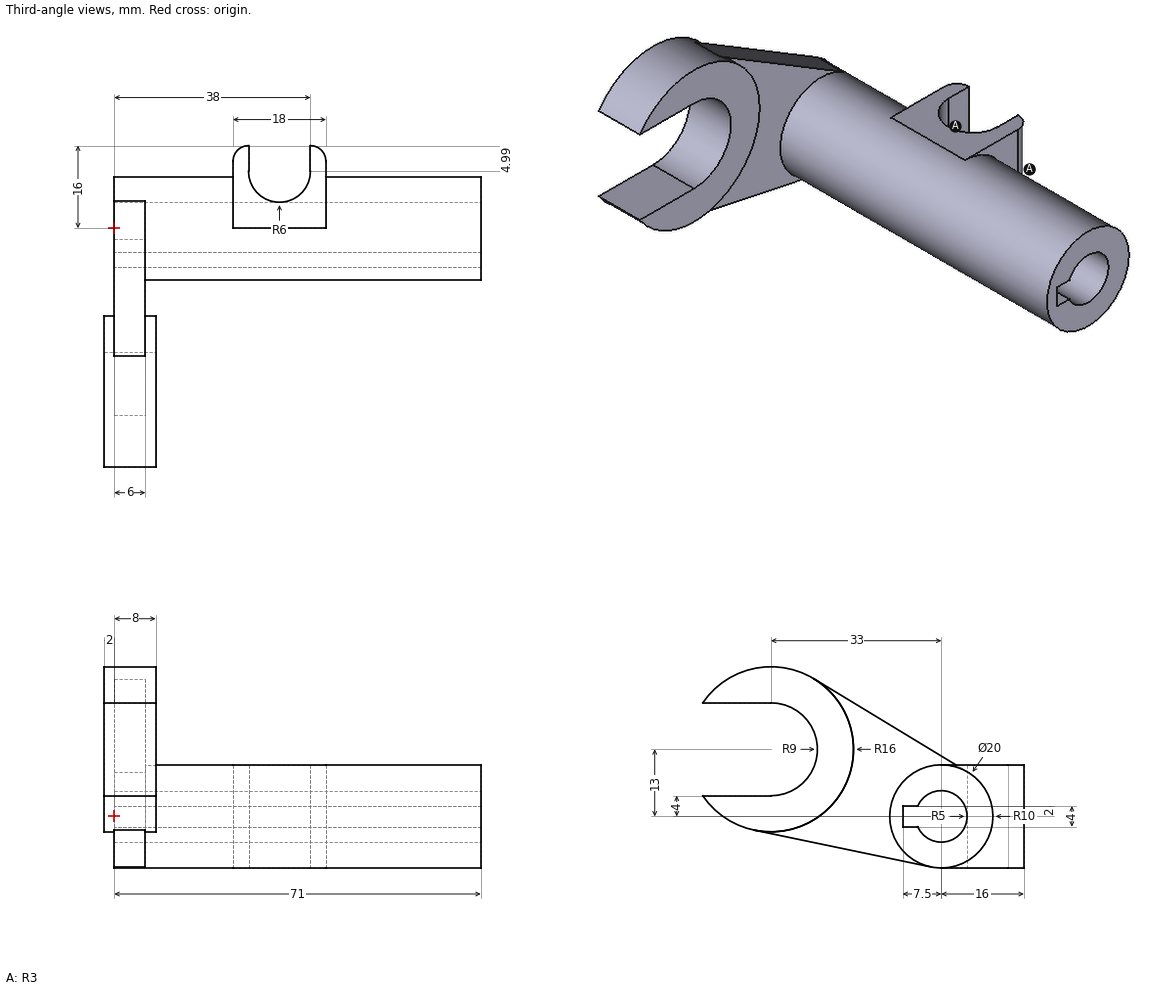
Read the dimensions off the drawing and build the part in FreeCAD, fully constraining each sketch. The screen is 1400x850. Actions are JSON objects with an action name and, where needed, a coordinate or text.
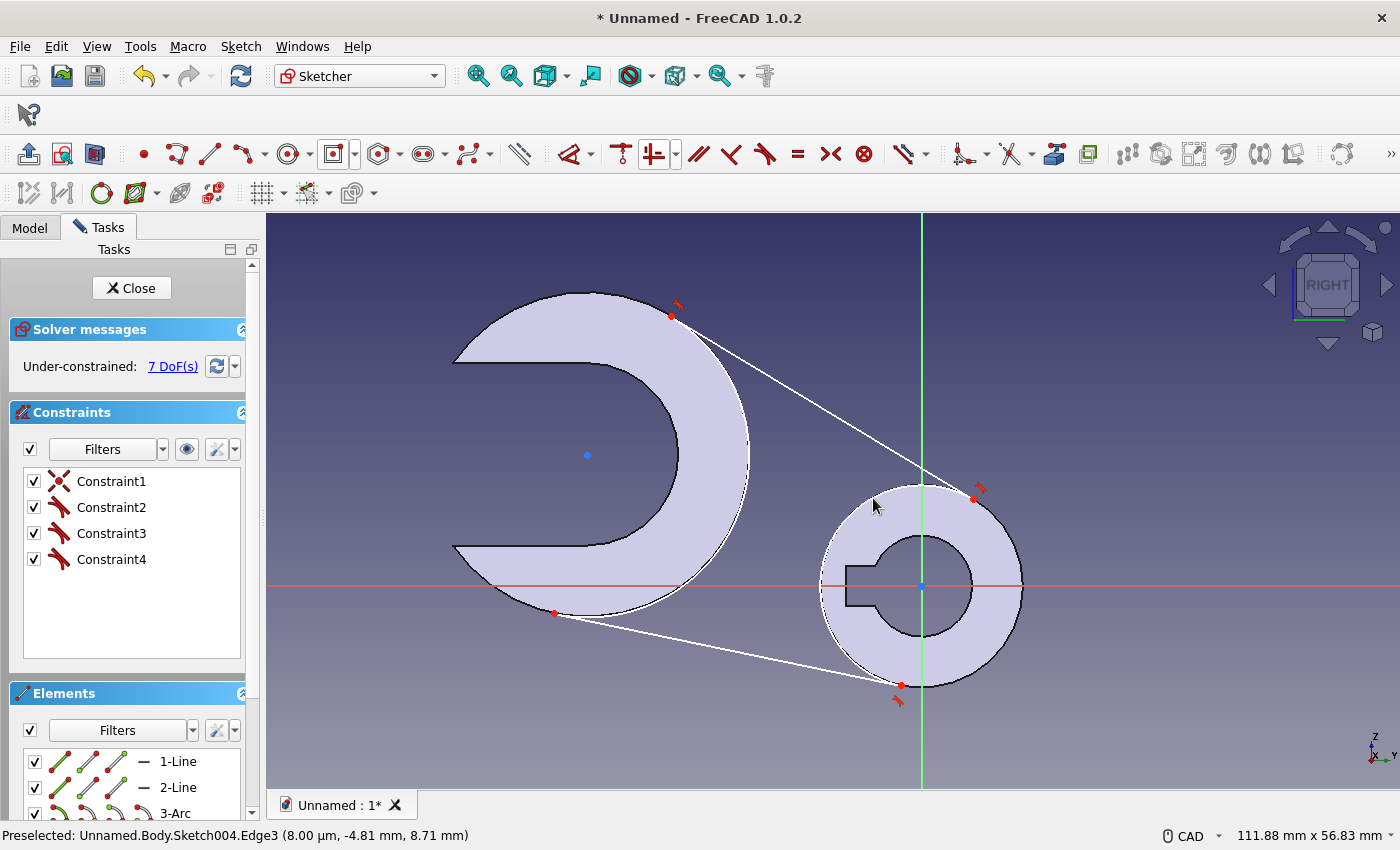
{"action": "left_click", "coordinate": [797, 664]}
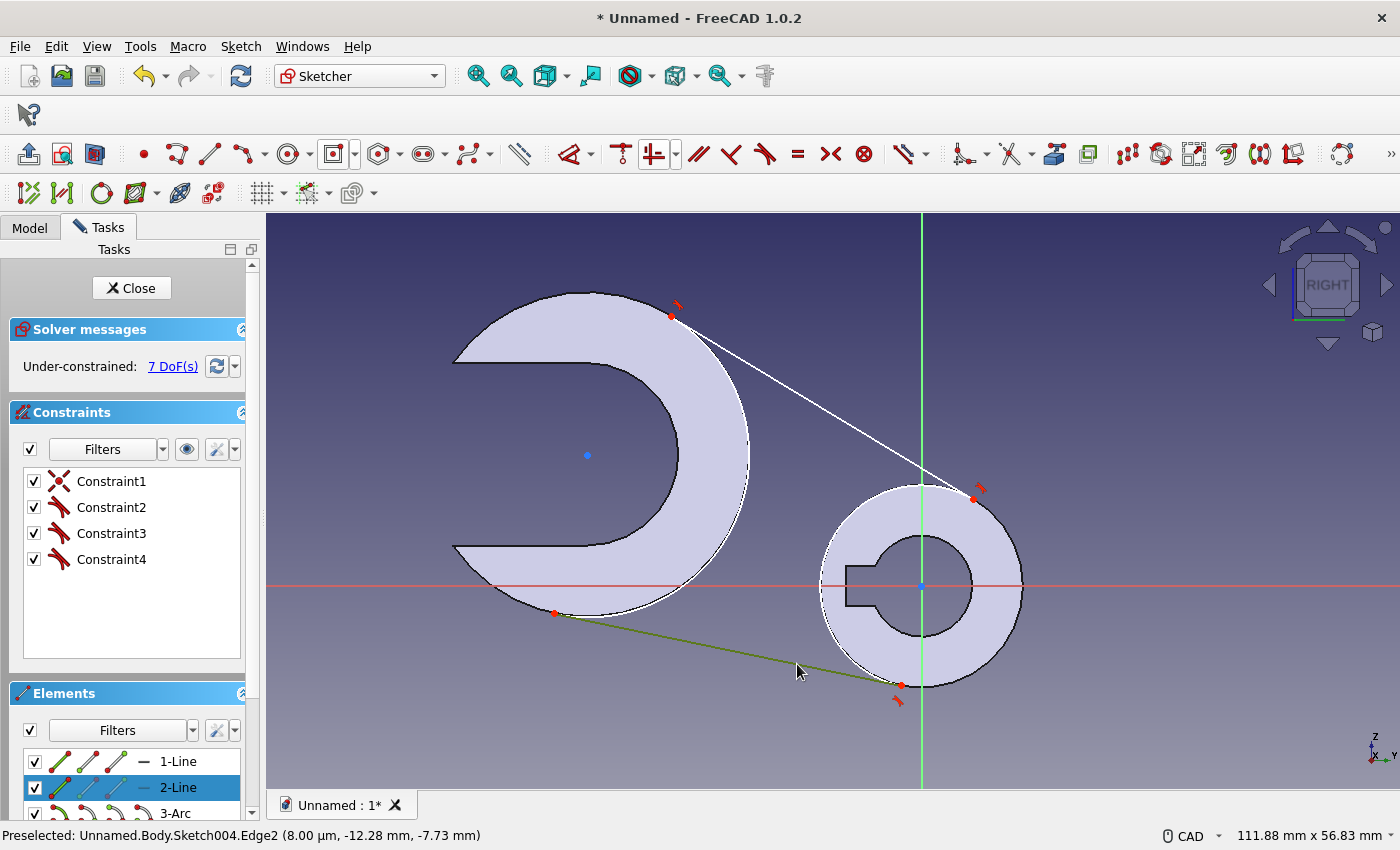
{"action": "left_click", "coordinate": [683, 586]}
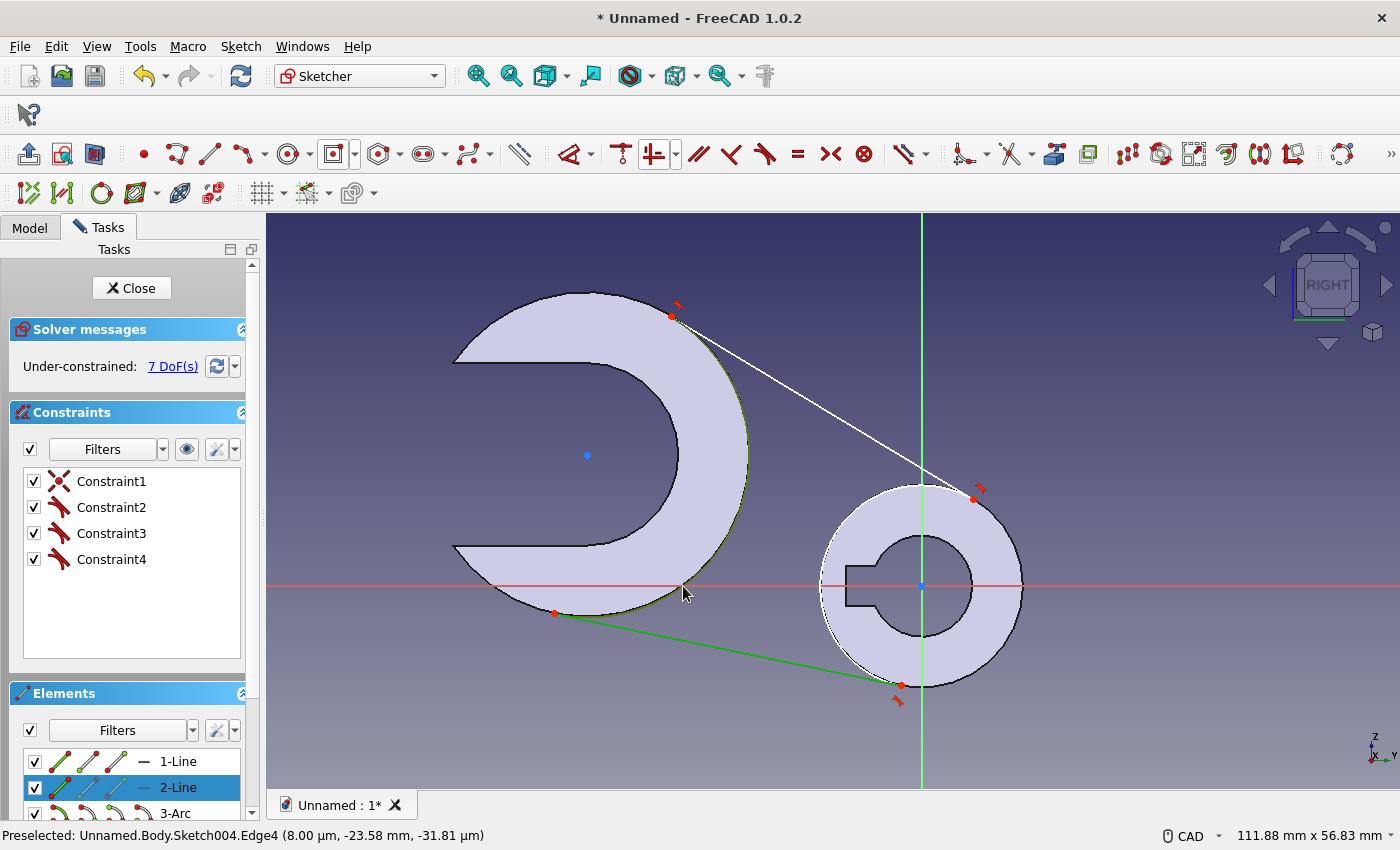
{"action": "key", "text": "t"}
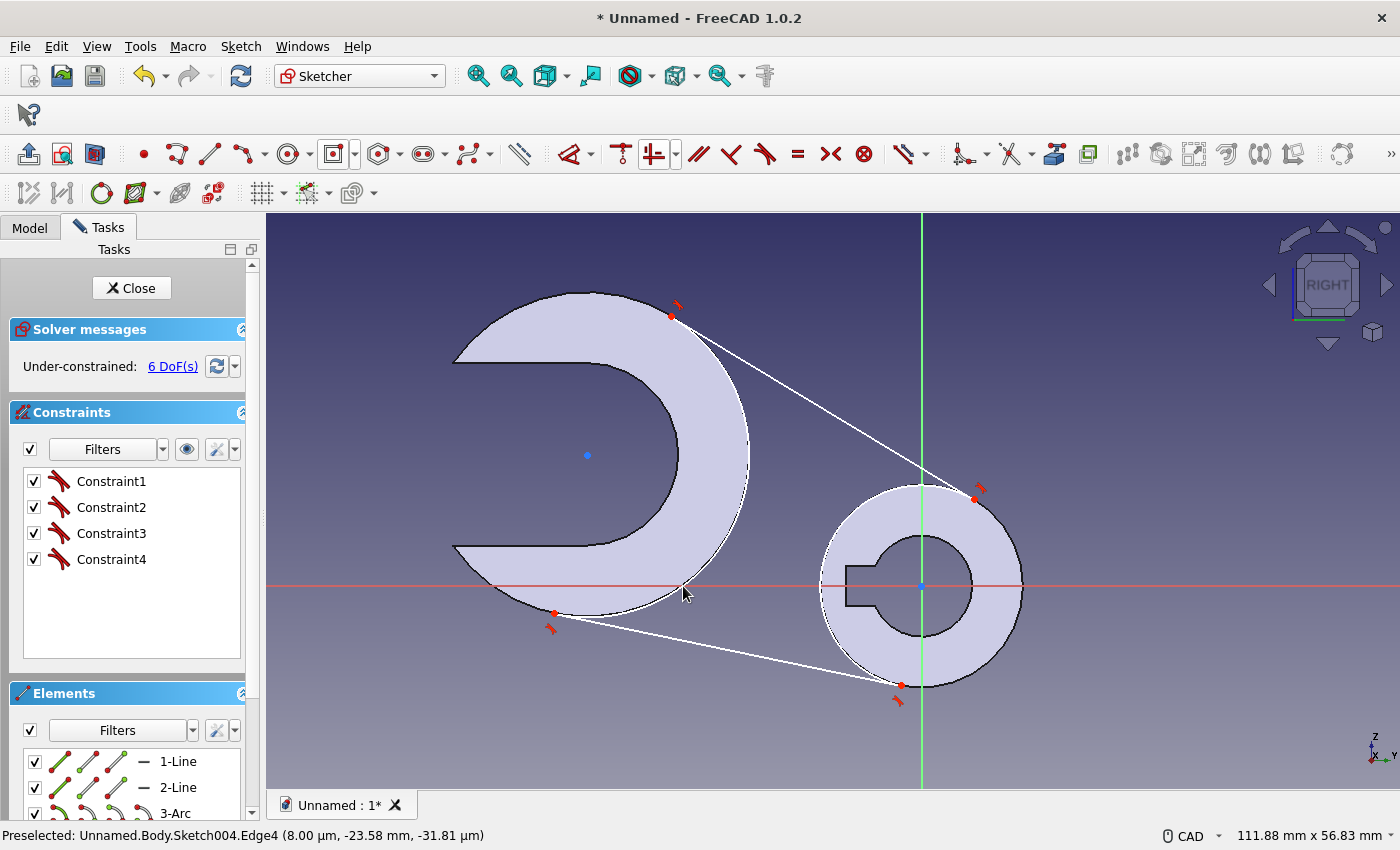
{"action": "left_click_drag", "start_coordinate": [912, 576], "coordinate": [932, 597]}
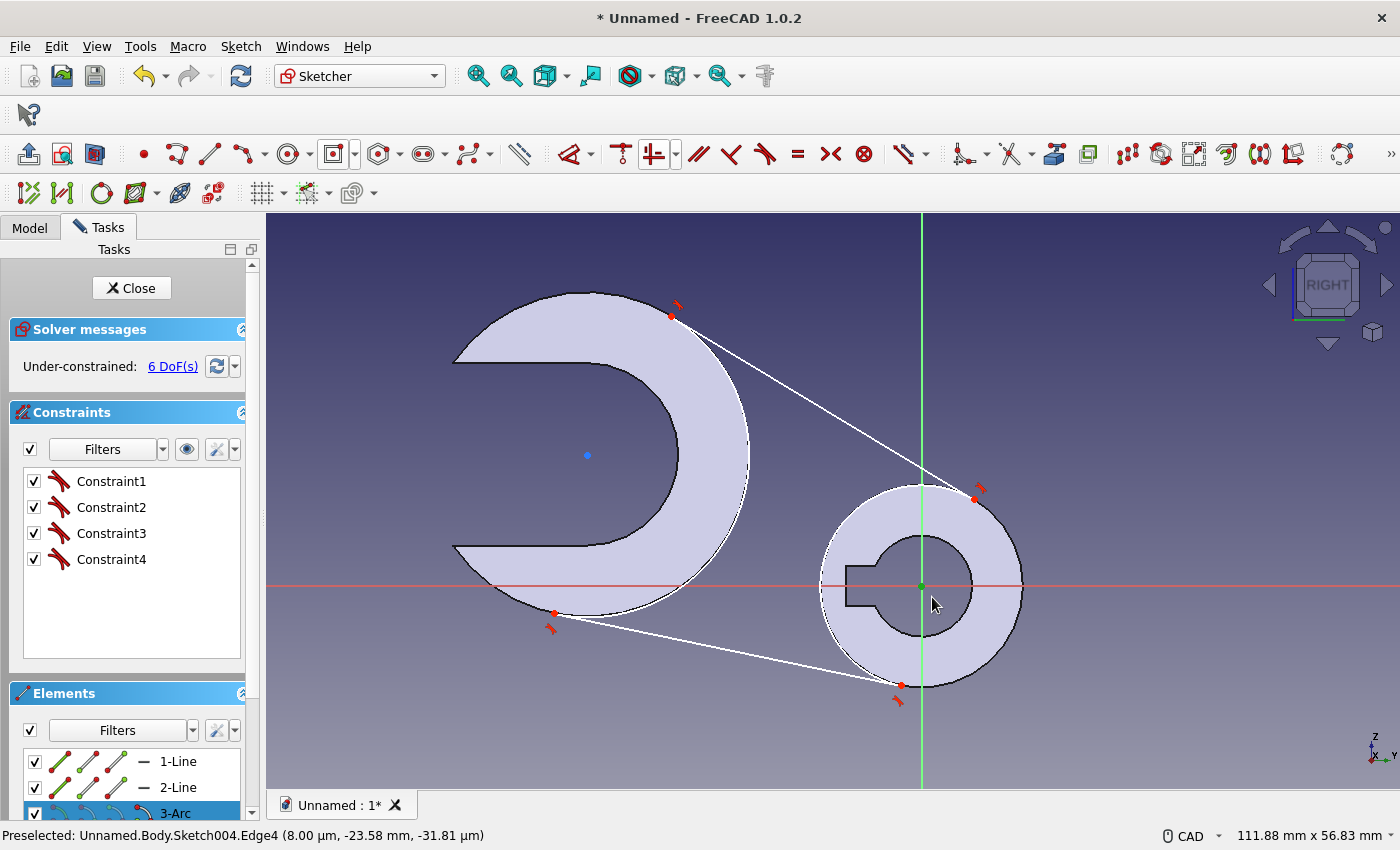
{"action": "key", "text": "c"}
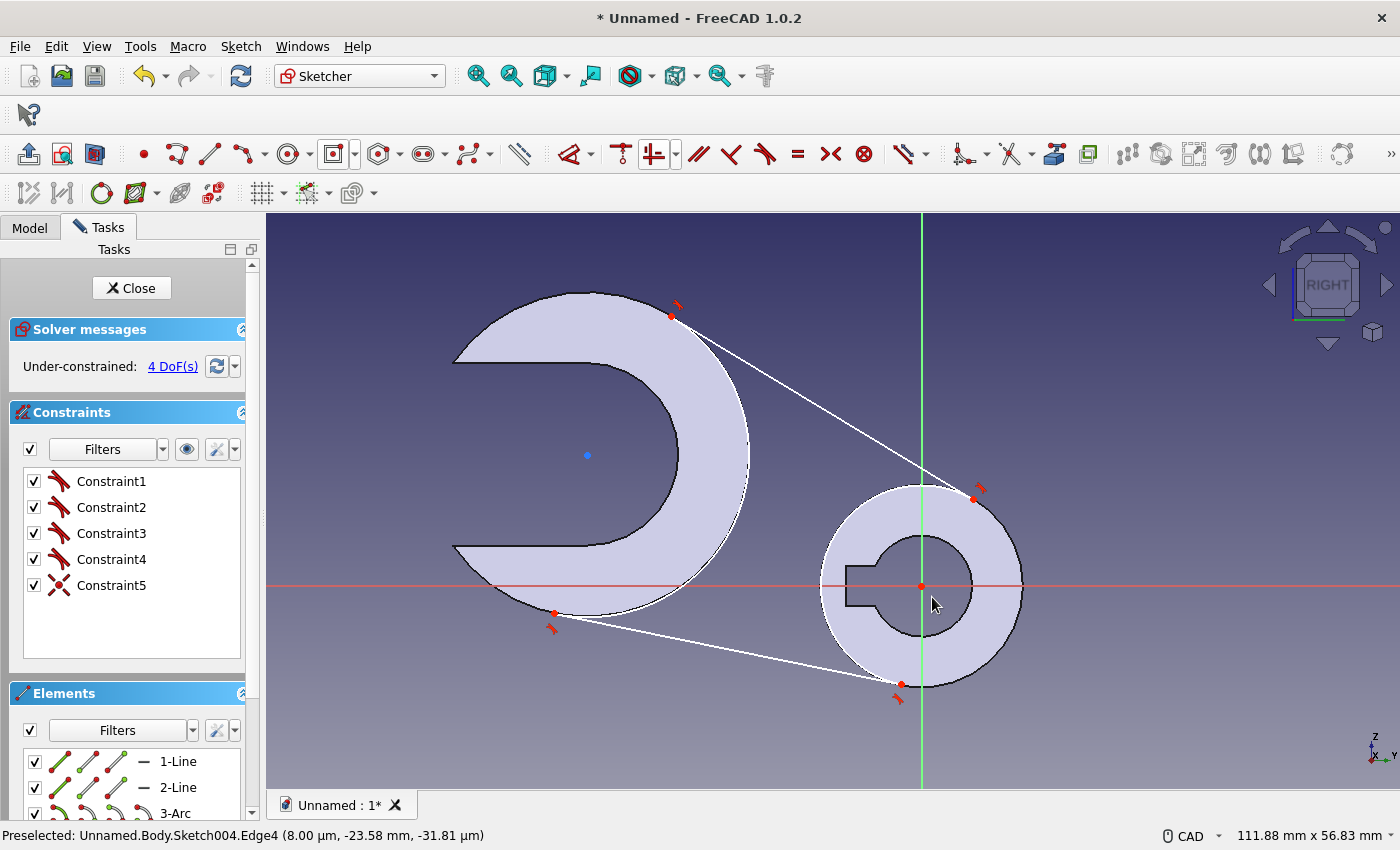
{"action": "key", "text": "d"}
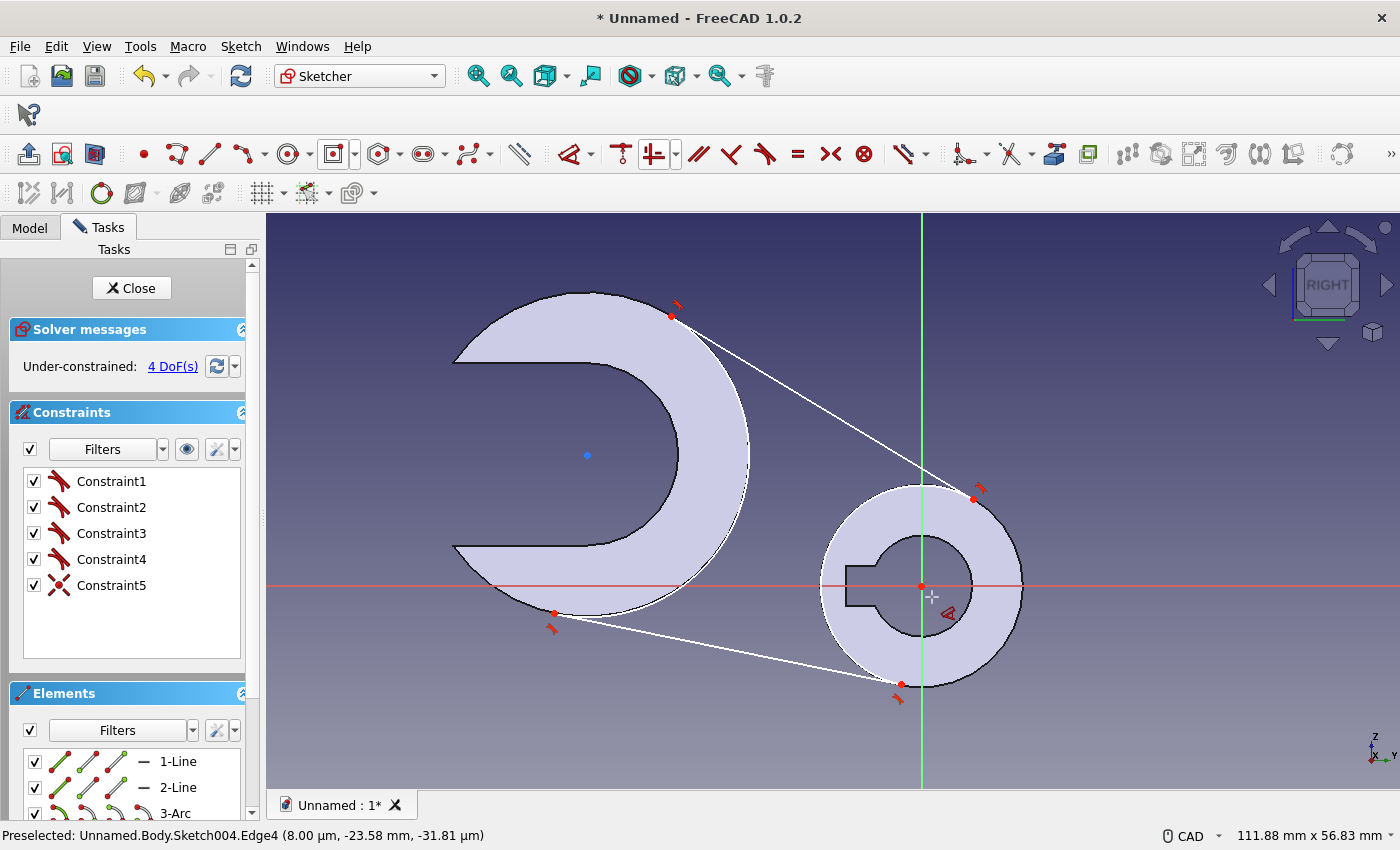
{"action": "left_click", "coordinate": [873, 498]}
{"action": "left_click", "coordinate": [858, 470]}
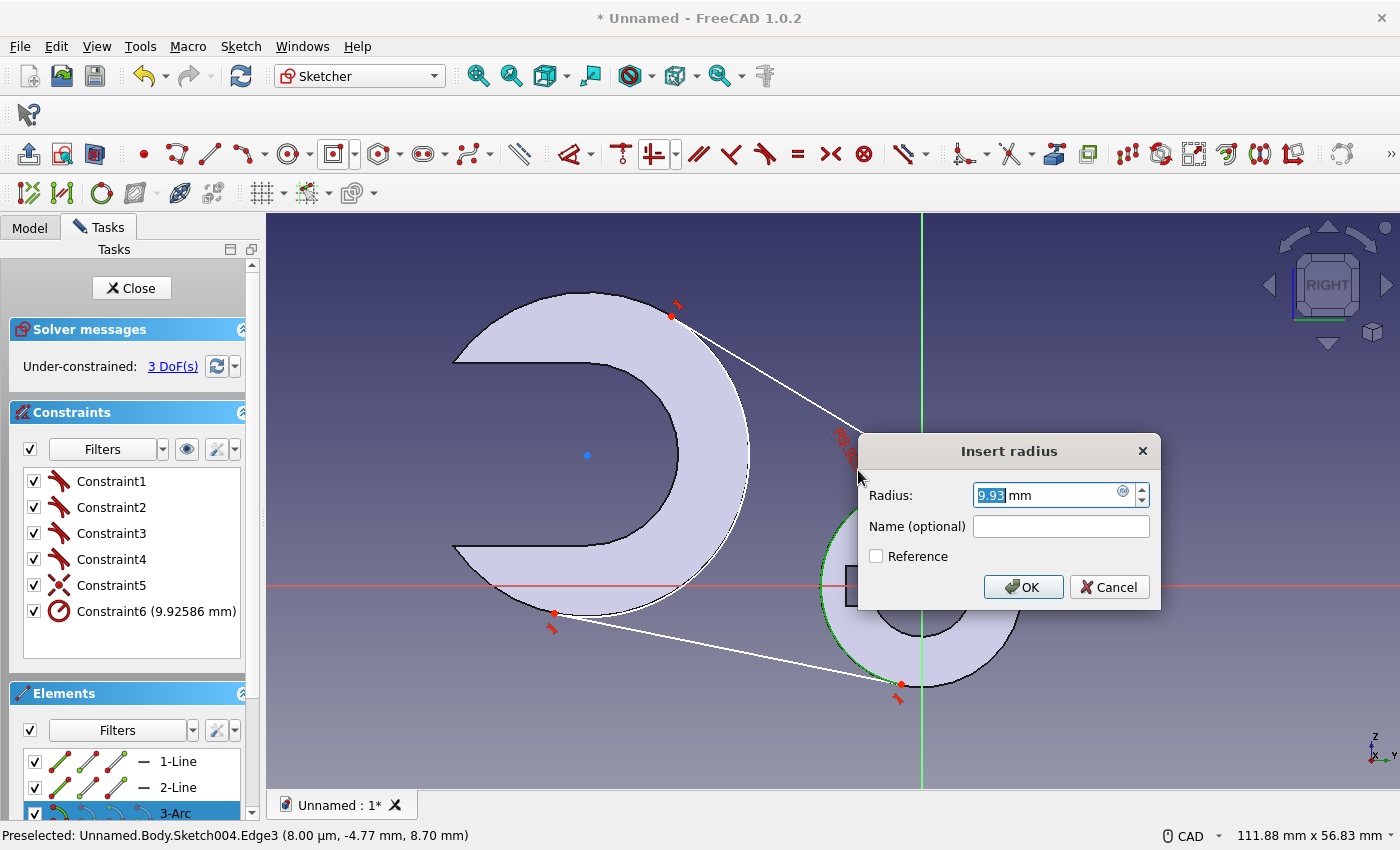
{"action": "type", "text": "10"}
{"action": "key", "text": "Return"}